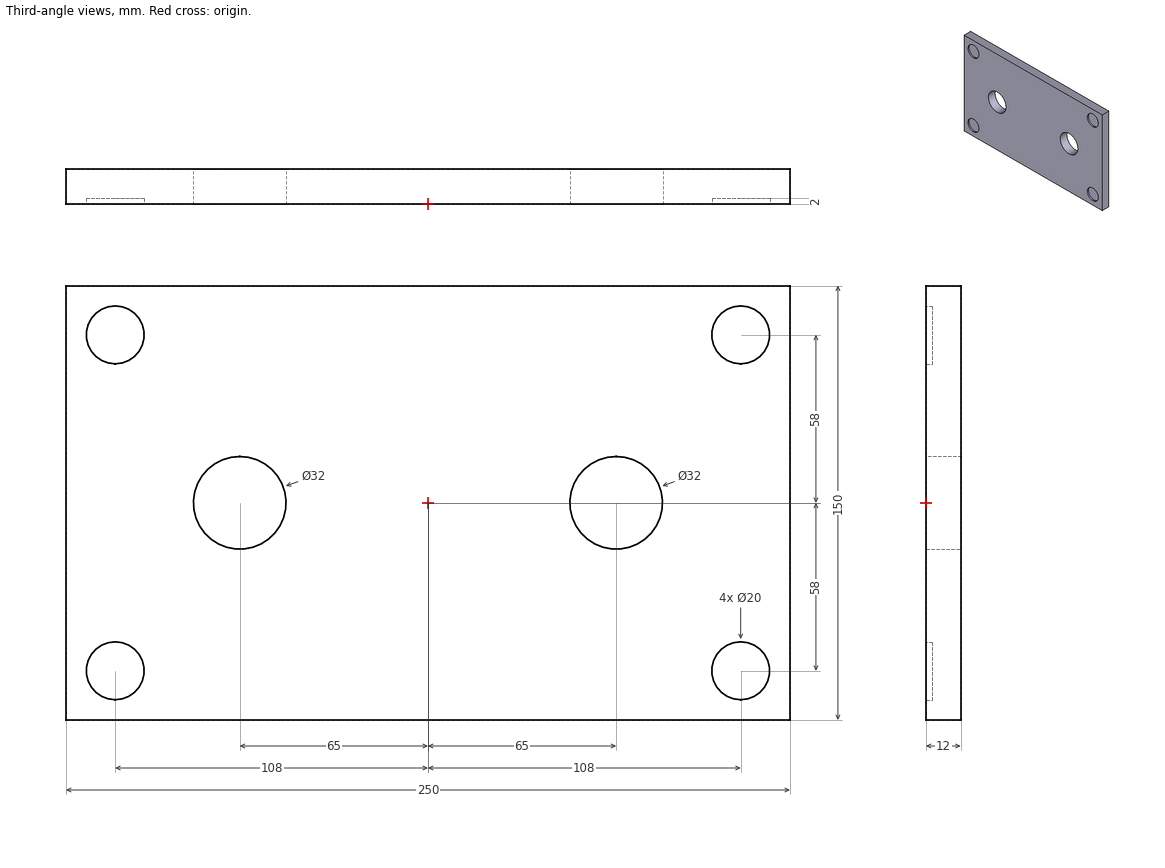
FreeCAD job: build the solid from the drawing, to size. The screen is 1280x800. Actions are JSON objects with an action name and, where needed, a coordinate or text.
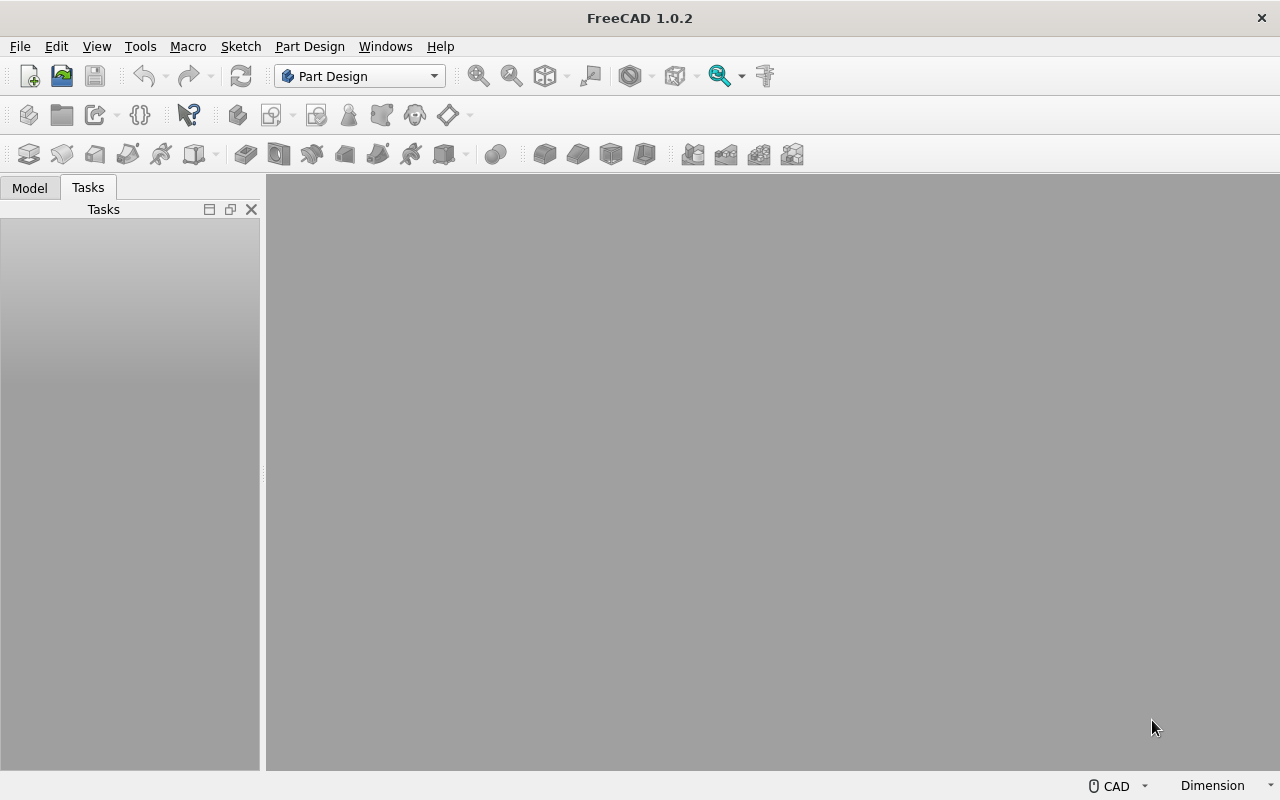
{"action": "left_click", "coordinate": [29, 76]}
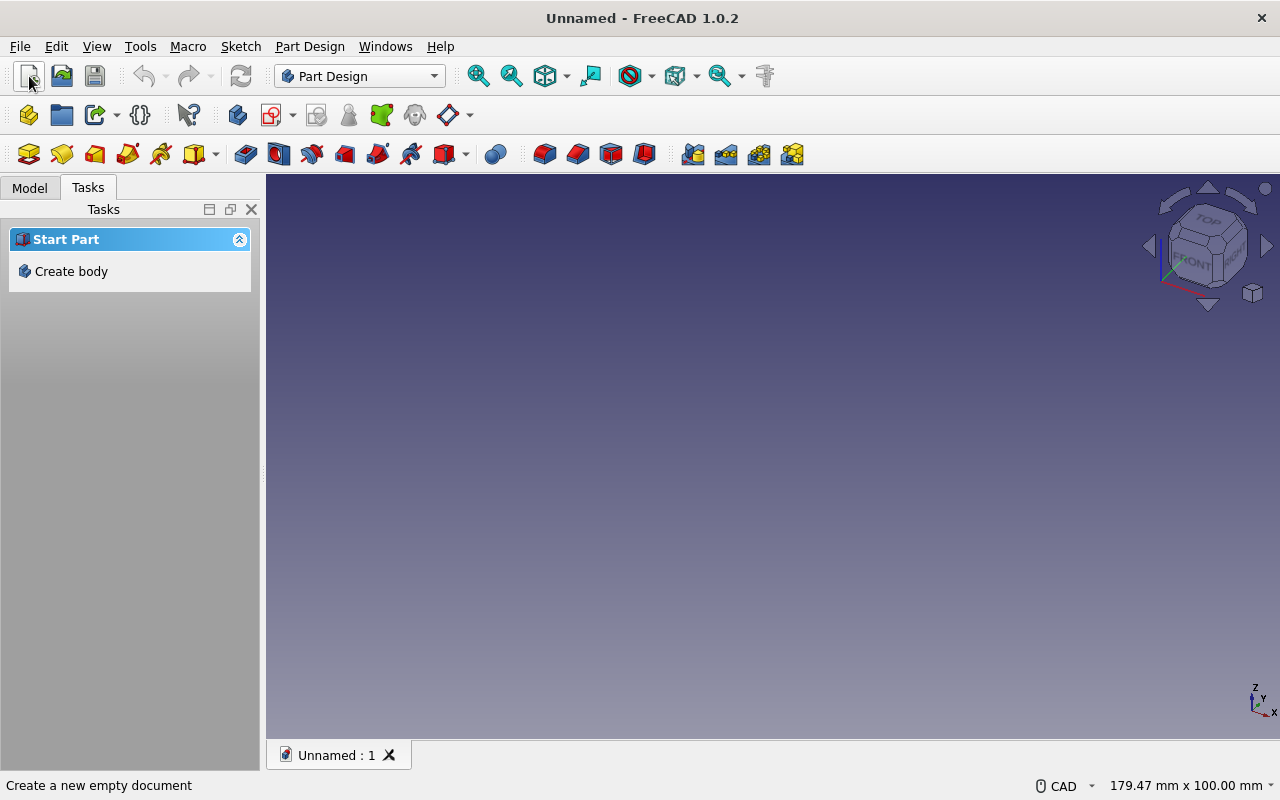
{"action": "left_click", "coordinate": [270, 116]}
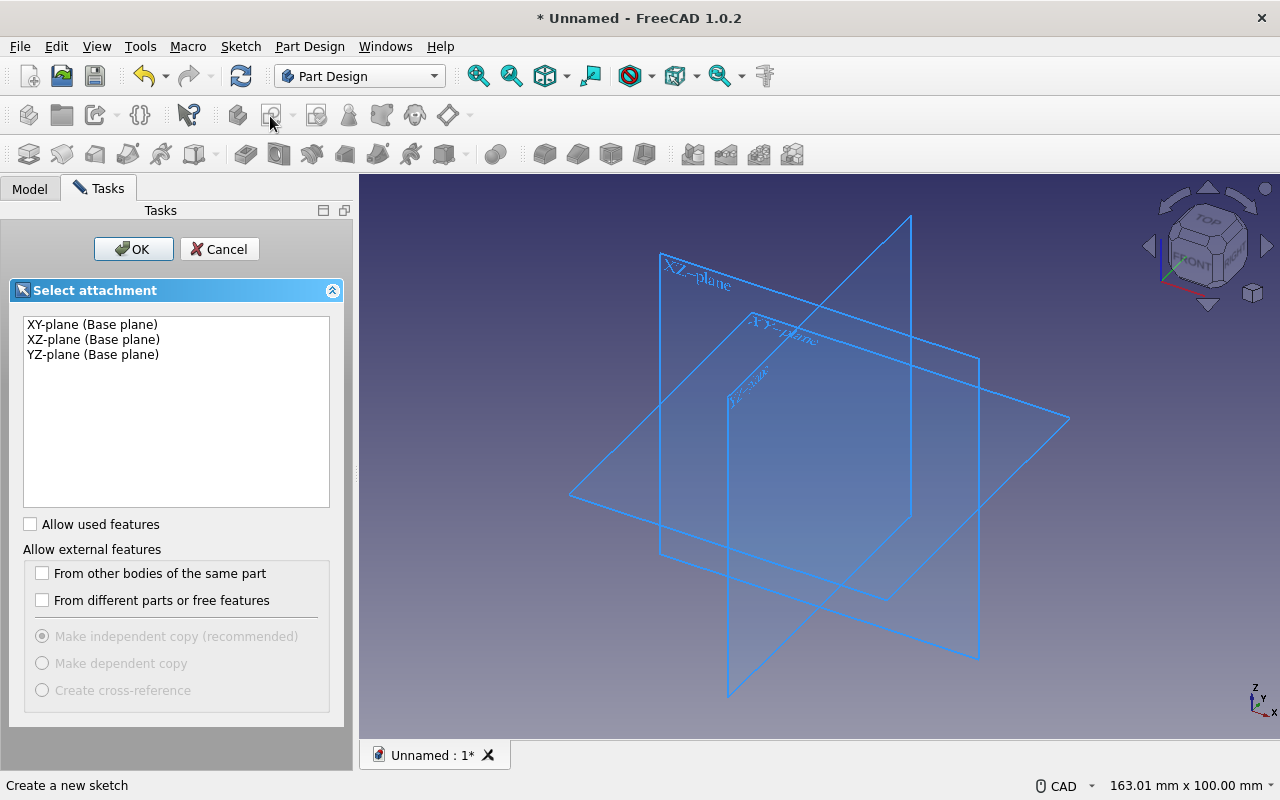
{"action": "left_click", "coordinate": [84, 340]}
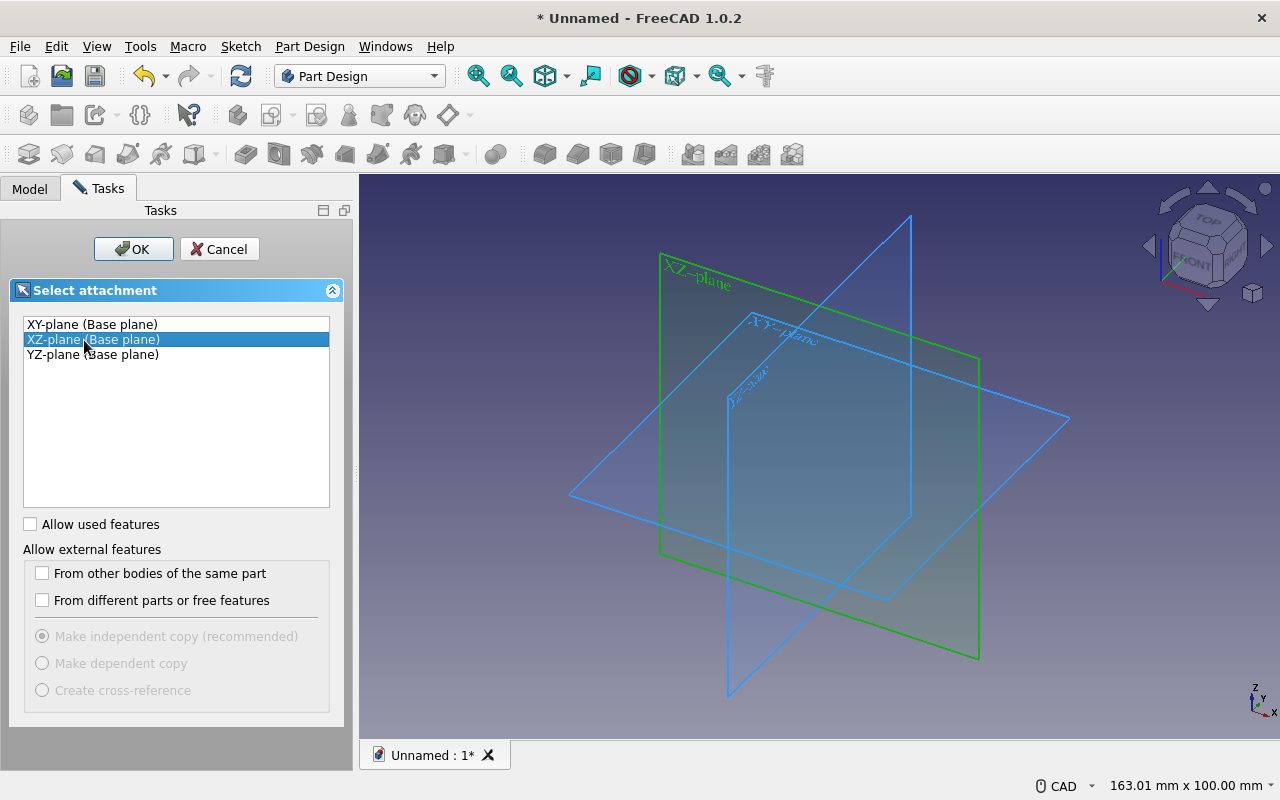
{"action": "left_click", "coordinate": [134, 249]}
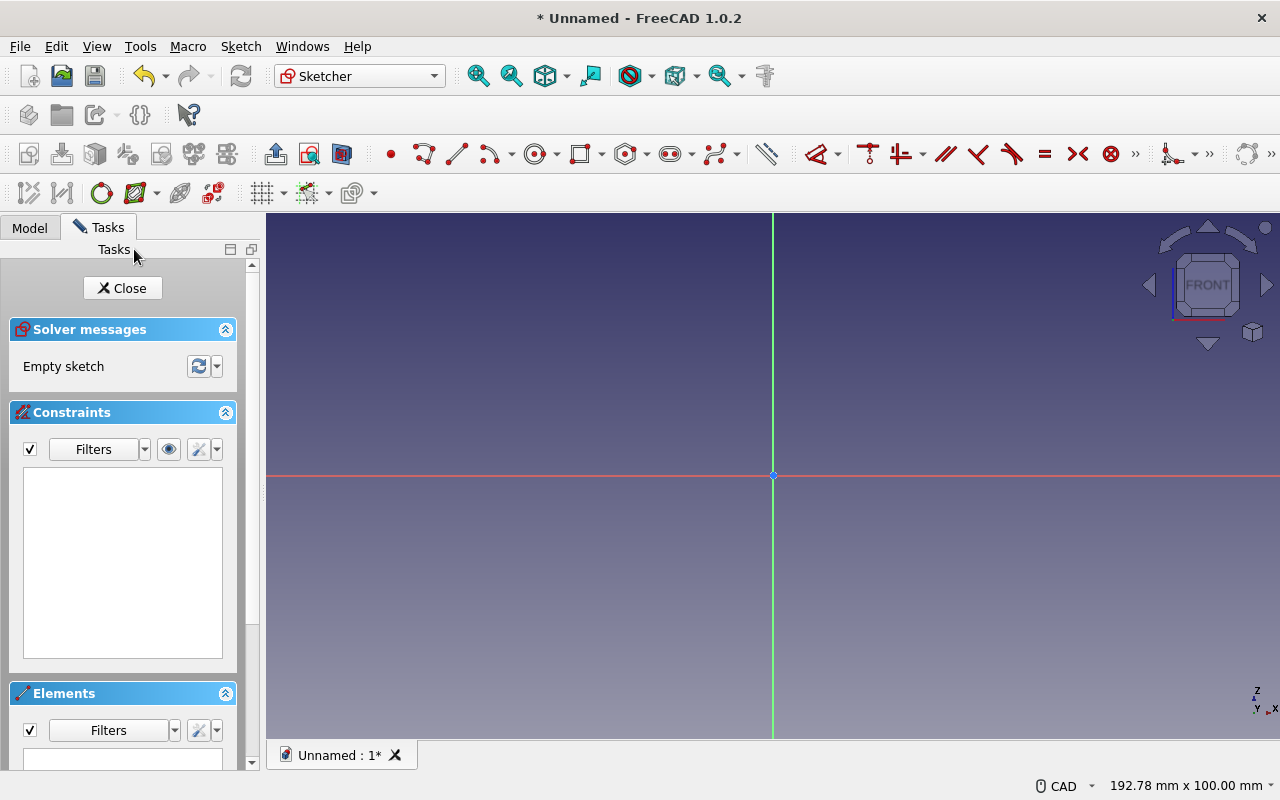
{"action": "scroll", "coordinate": [649, 476], "scroll_direction": "down", "scroll_amount": 4}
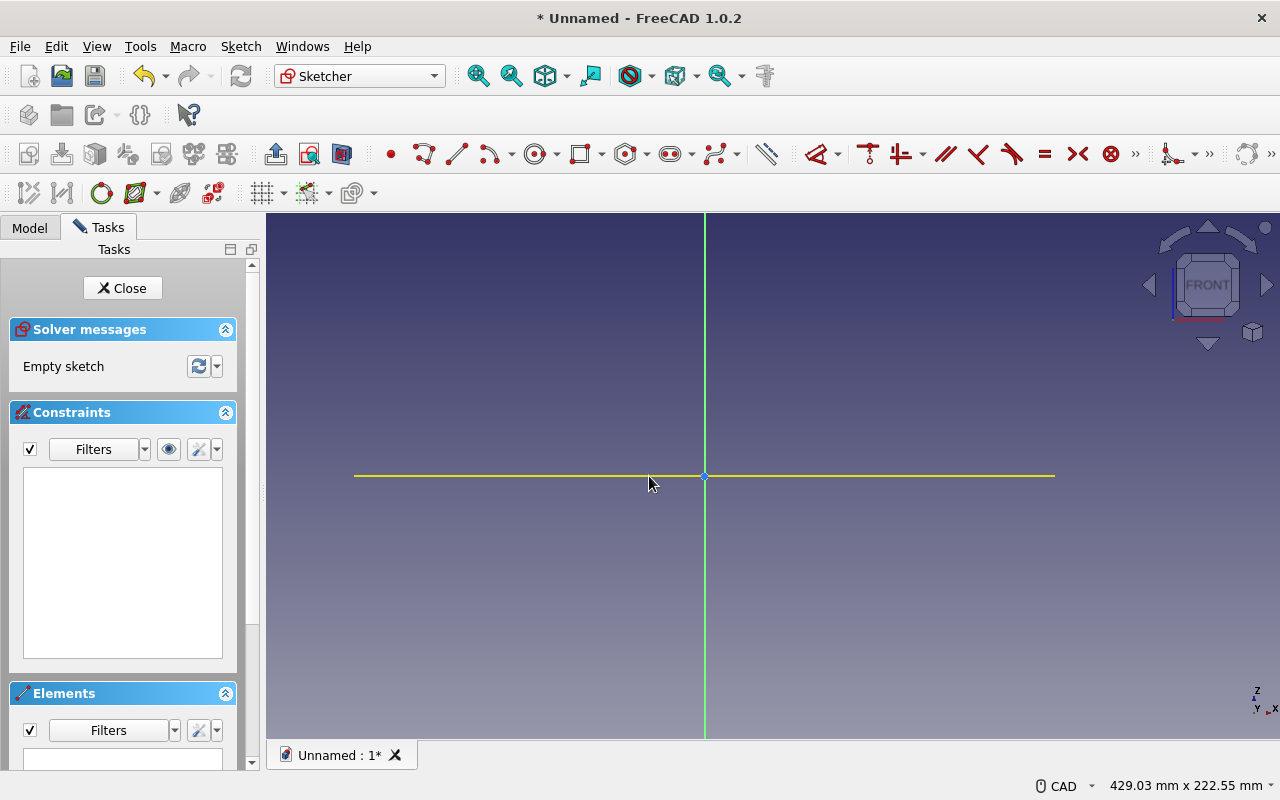
{"action": "key", "text": "g v"}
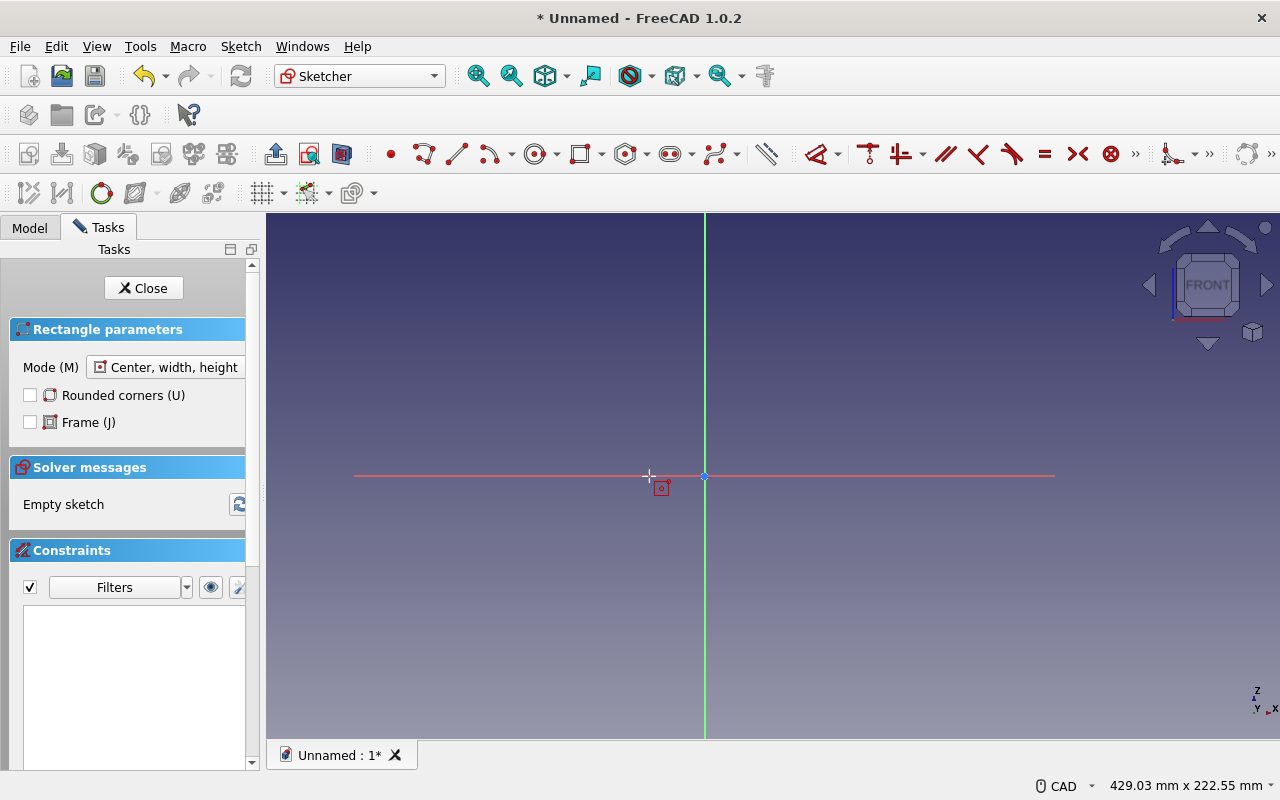
{"action": "left_click", "coordinate": [705, 476]}
{"action": "mouse_move", "coordinate": [1000, 299]}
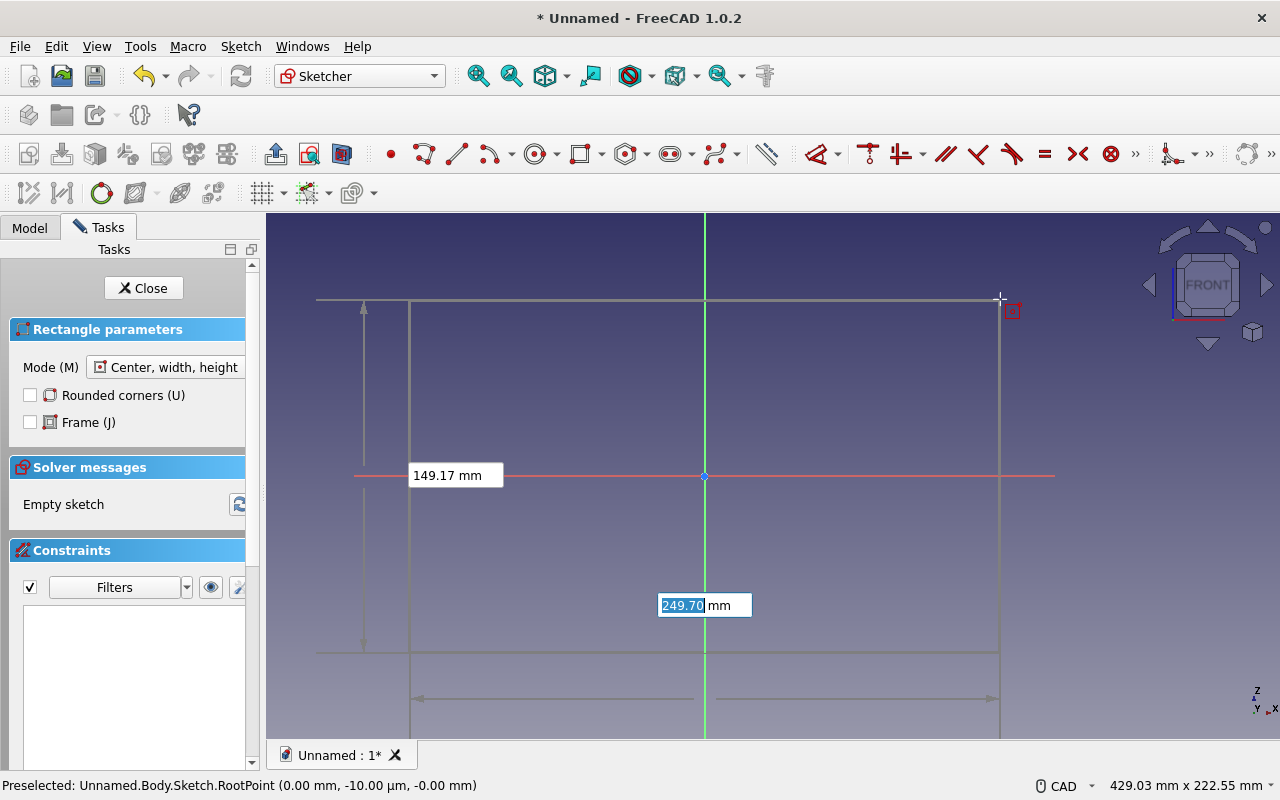
{"action": "type", "text": "250"}
{"action": "key", "text": "Tab"}
{"action": "type", "text": "150"}
{"action": "key", "text": "Return"}
{"action": "key", "text": "Escape"}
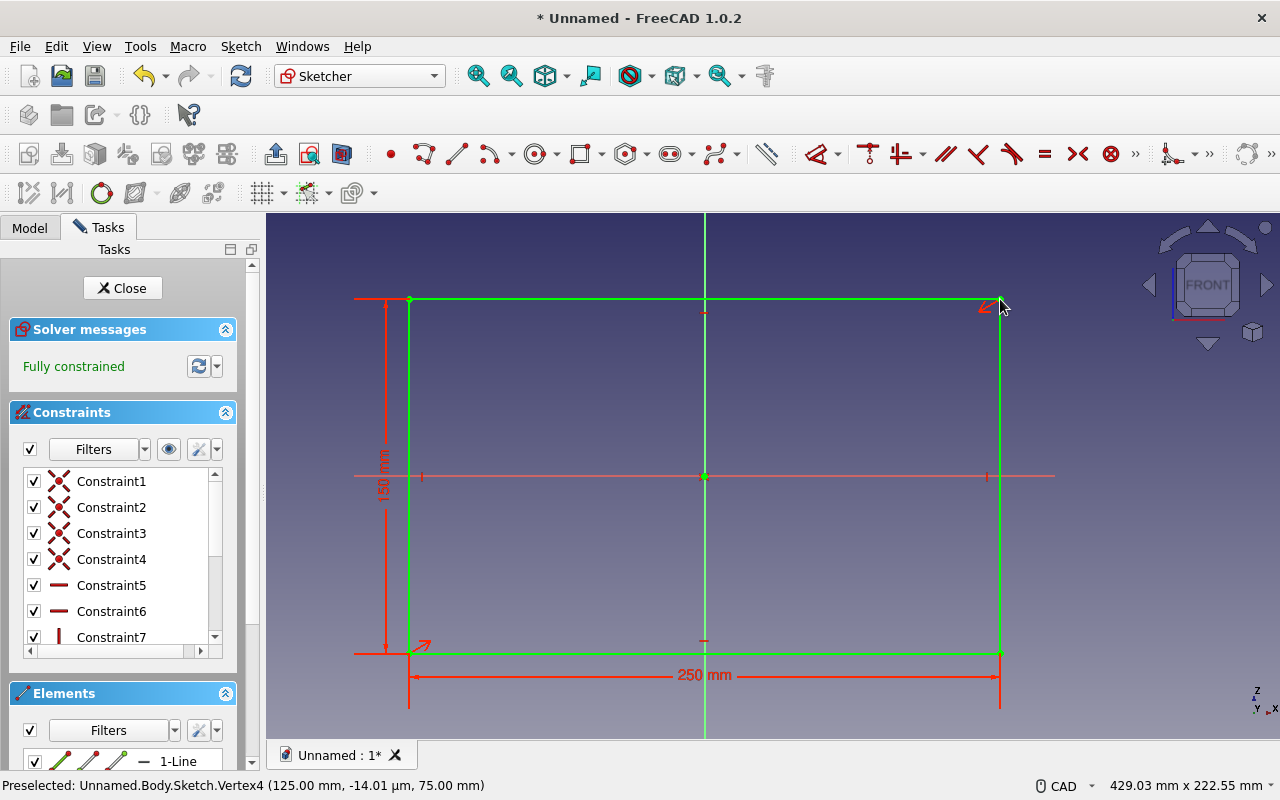
{"action": "left_click", "coordinate": [123, 288]}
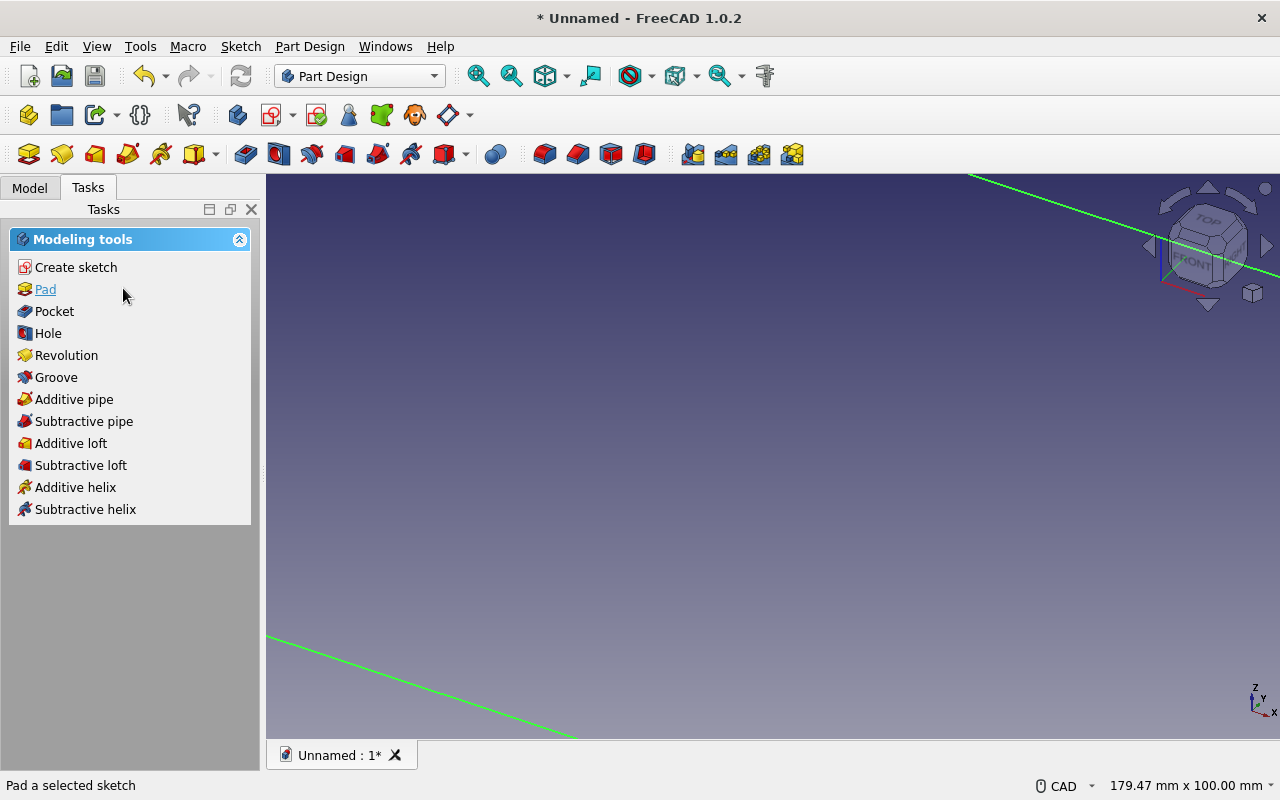
{"action": "left_click", "coordinate": [29, 154]}